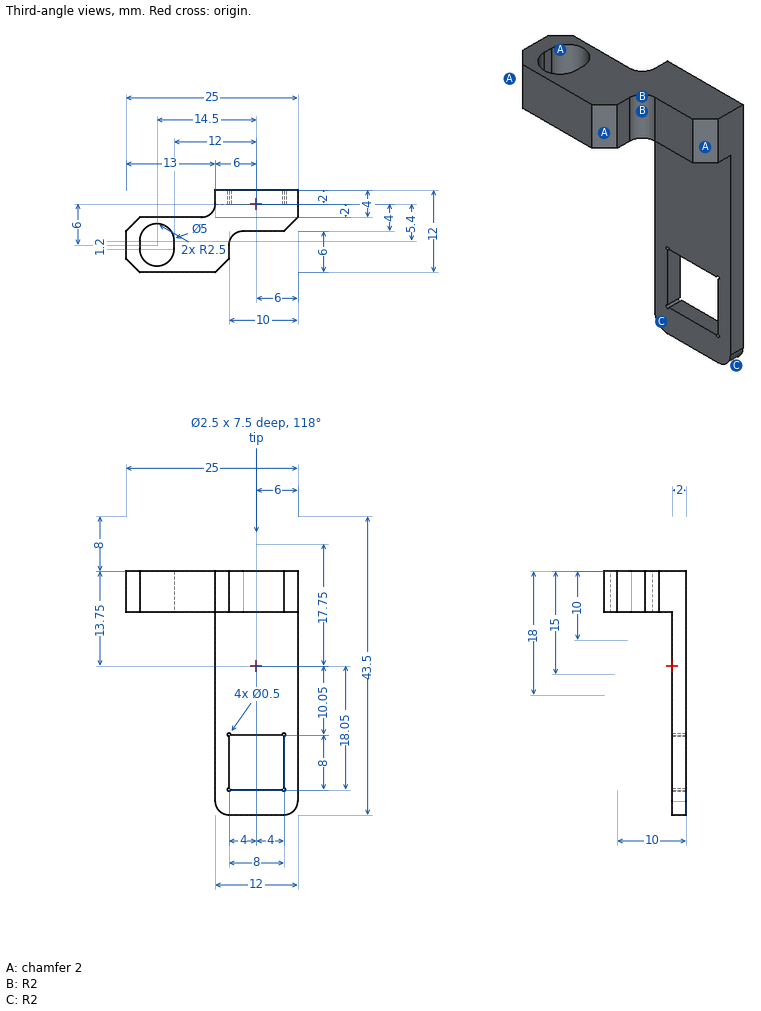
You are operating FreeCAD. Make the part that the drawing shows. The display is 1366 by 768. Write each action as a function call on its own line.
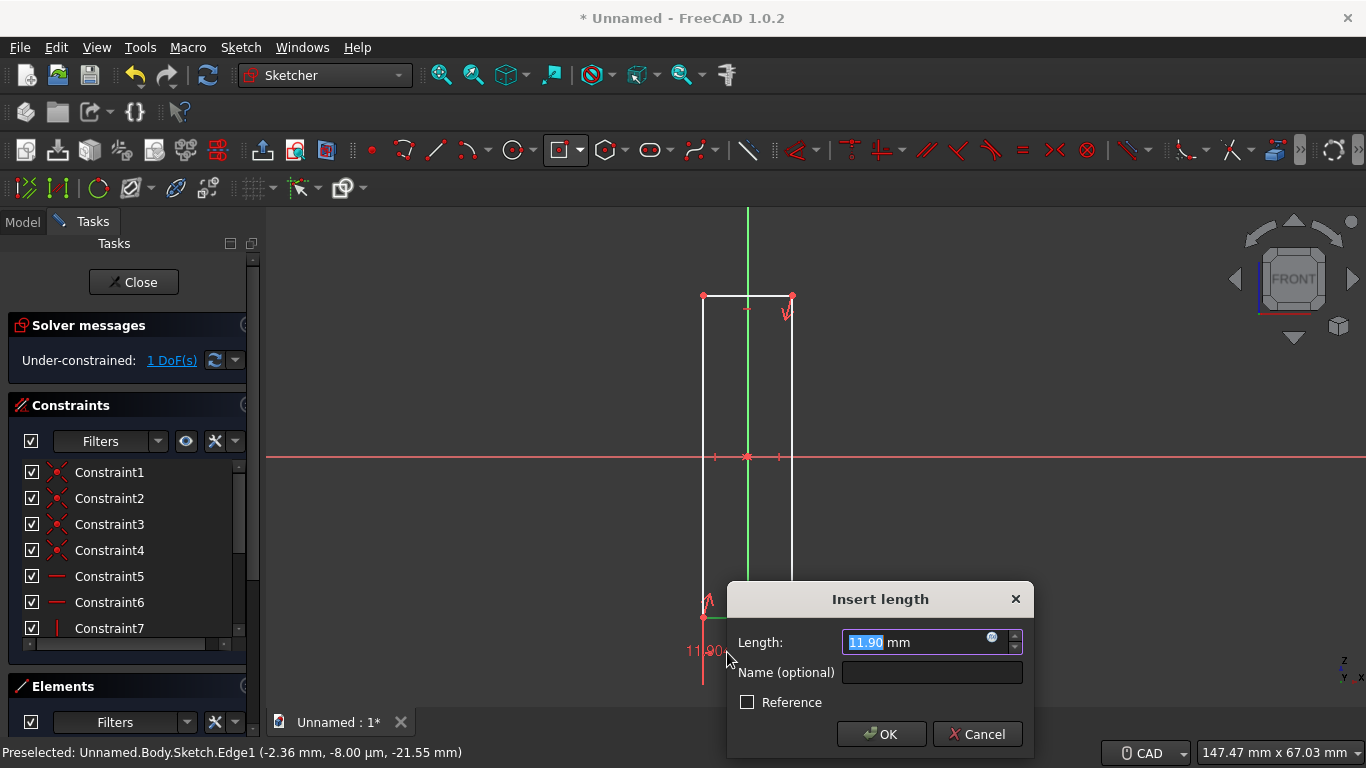
text(12)
key(Return)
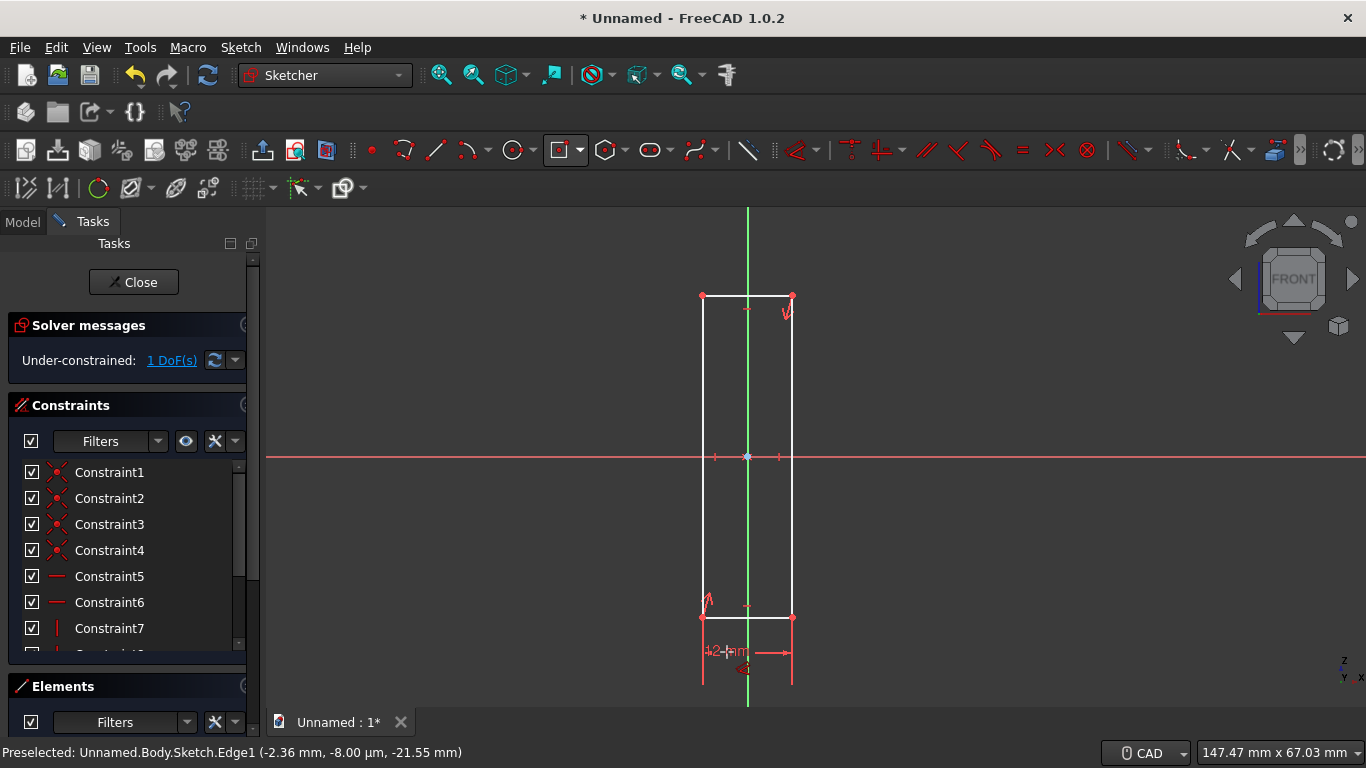
click(792, 521)
click(826, 383)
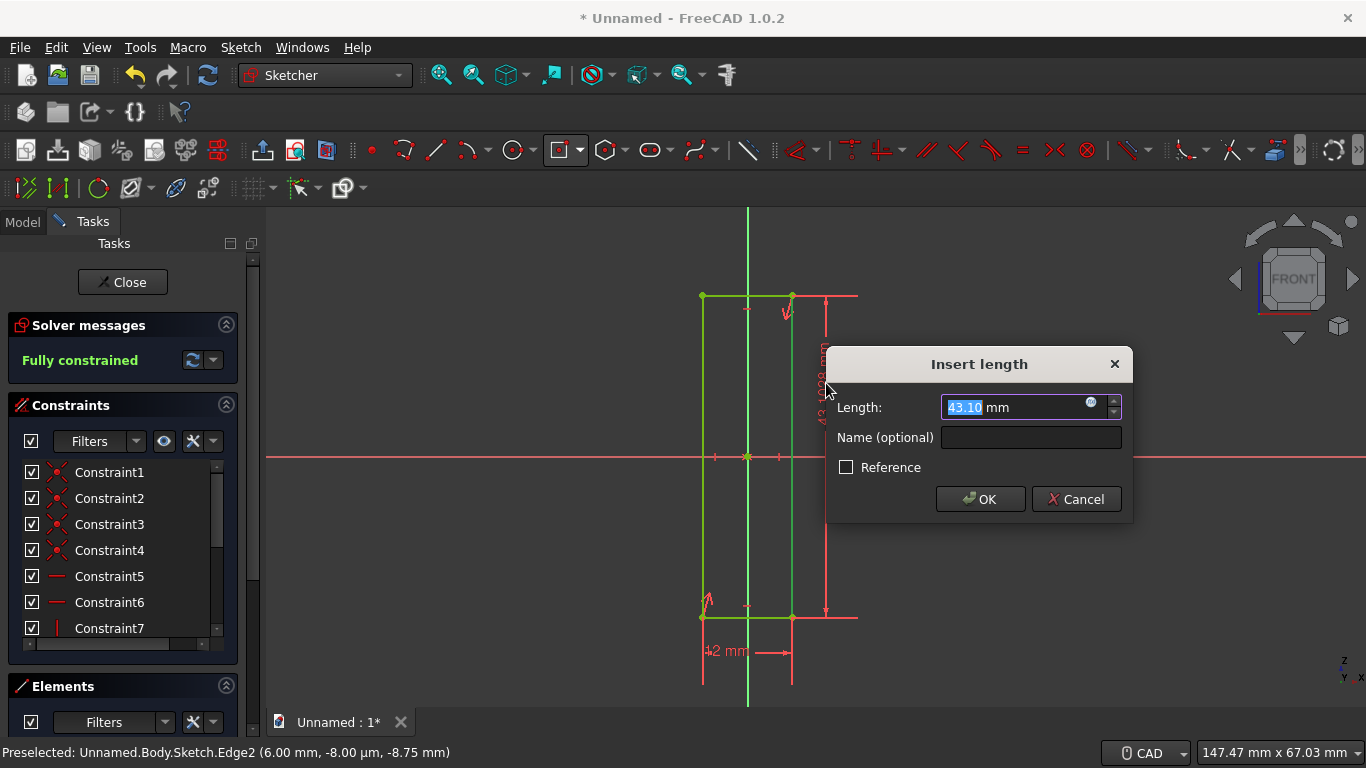
text(43.5)
key(Return)
key(Escape)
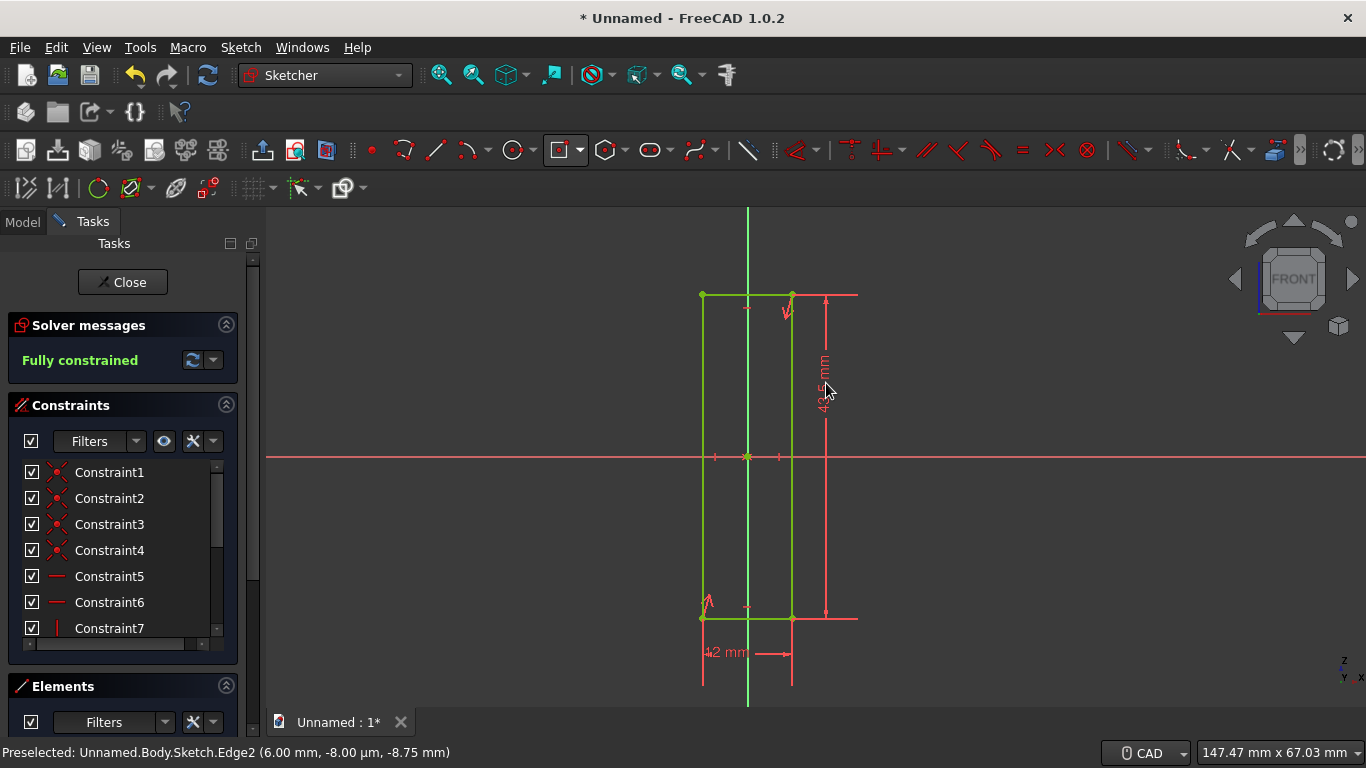
click(123, 282)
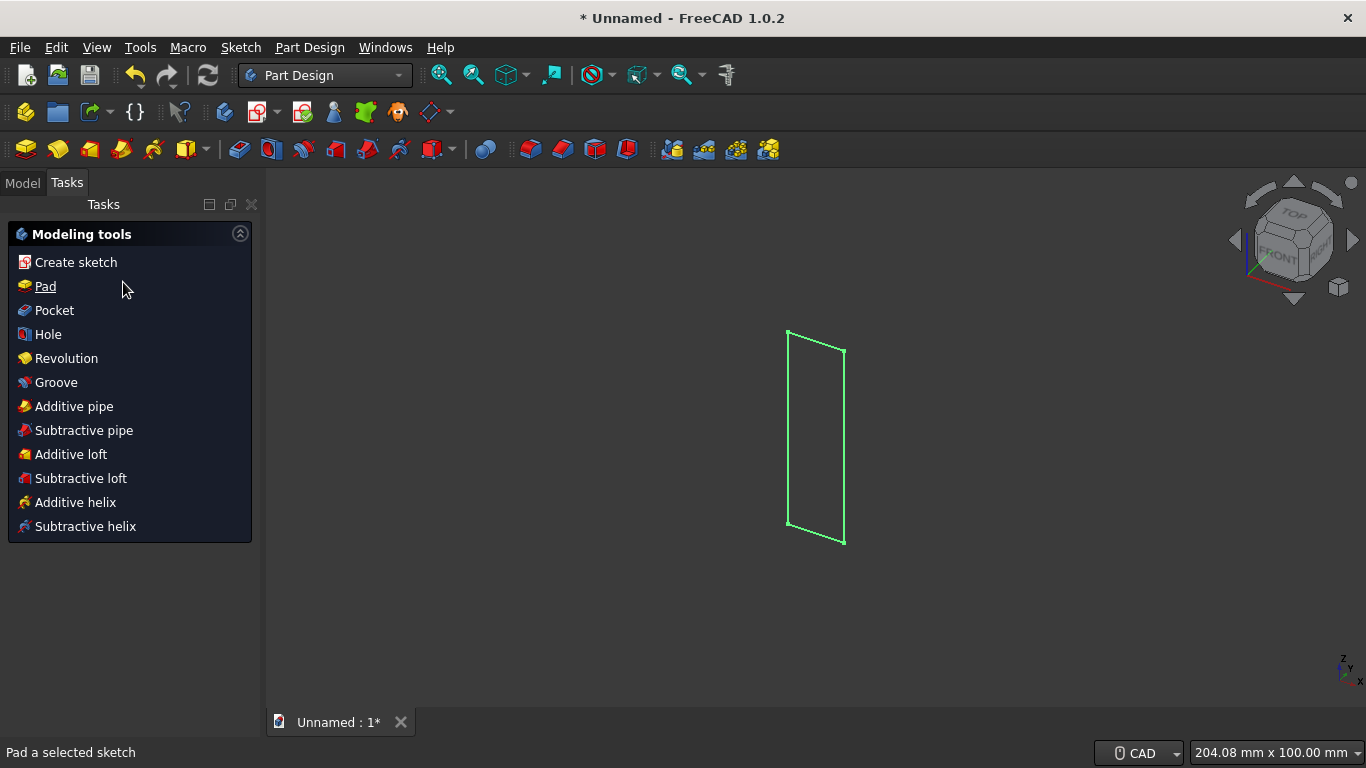
click(26, 150)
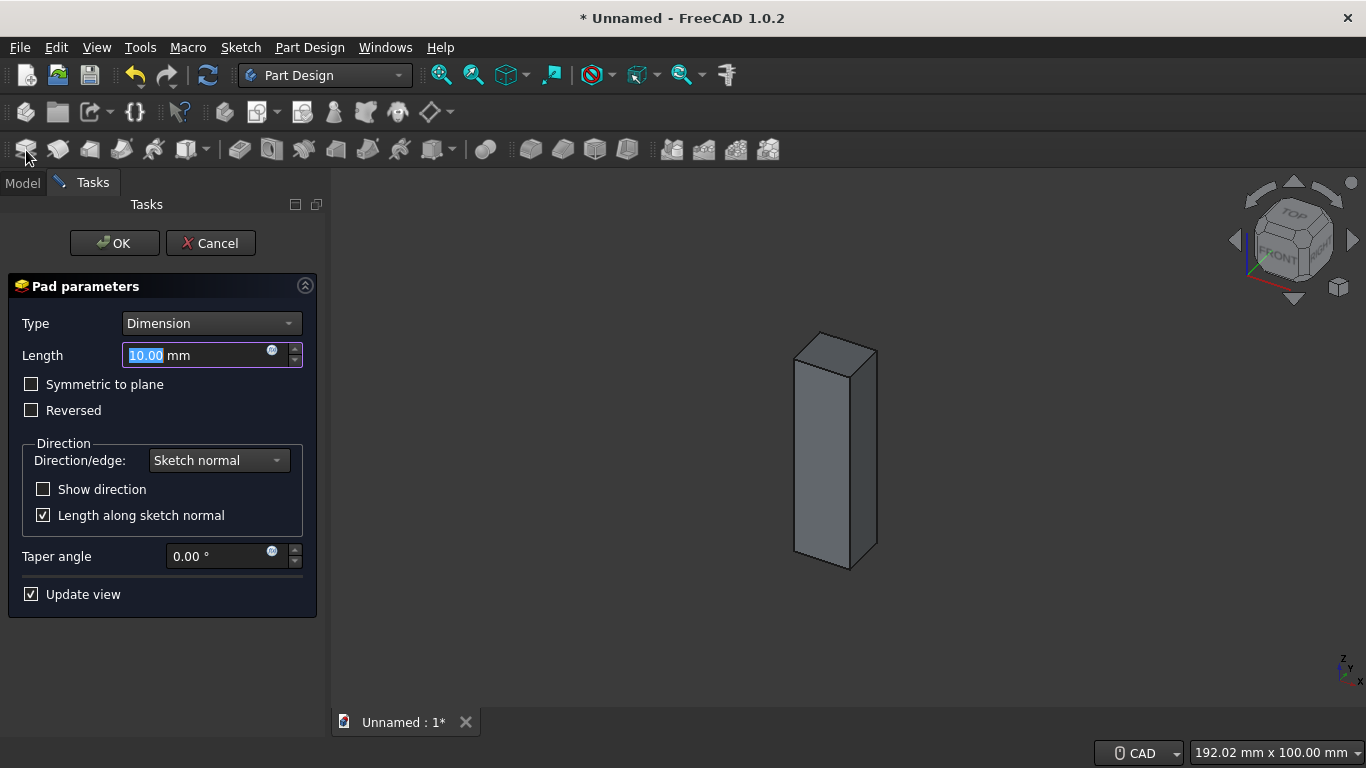
text(2)
key(Tab)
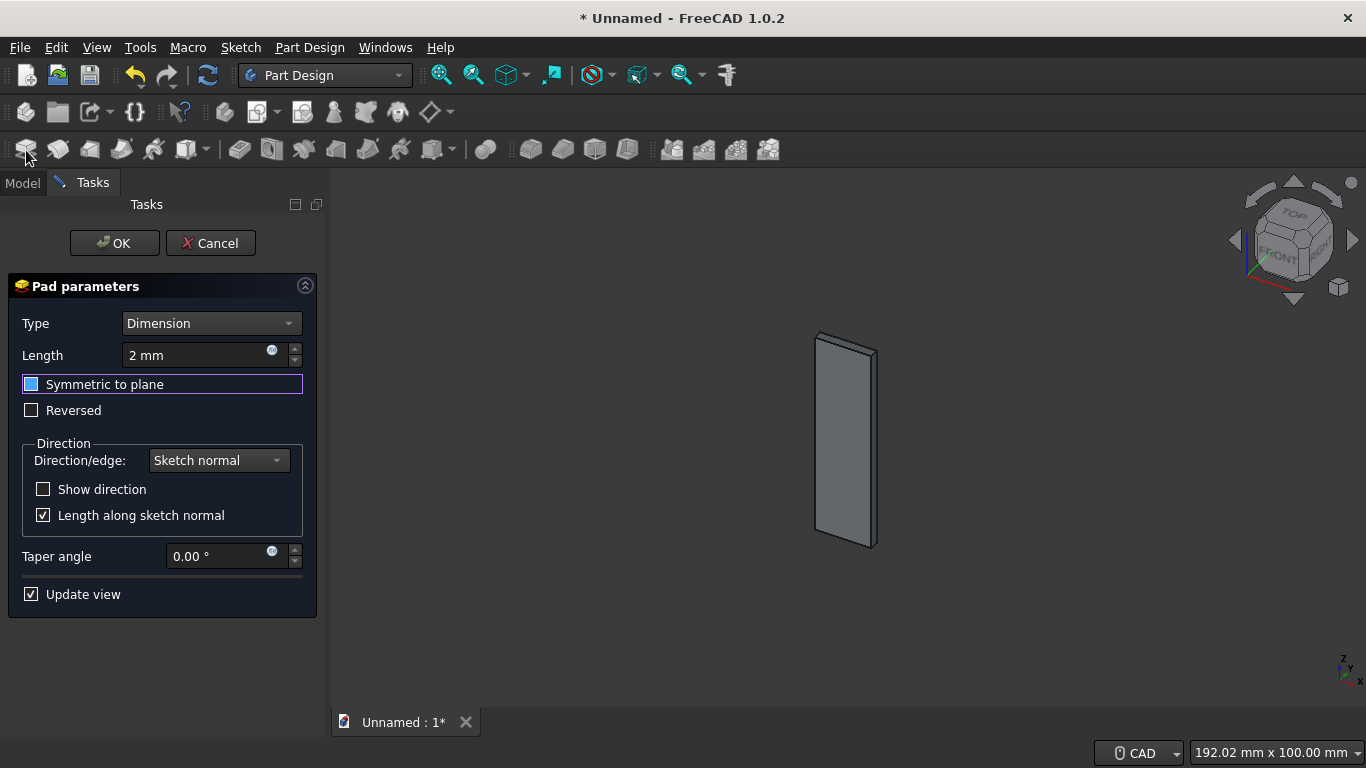
click(30, 410)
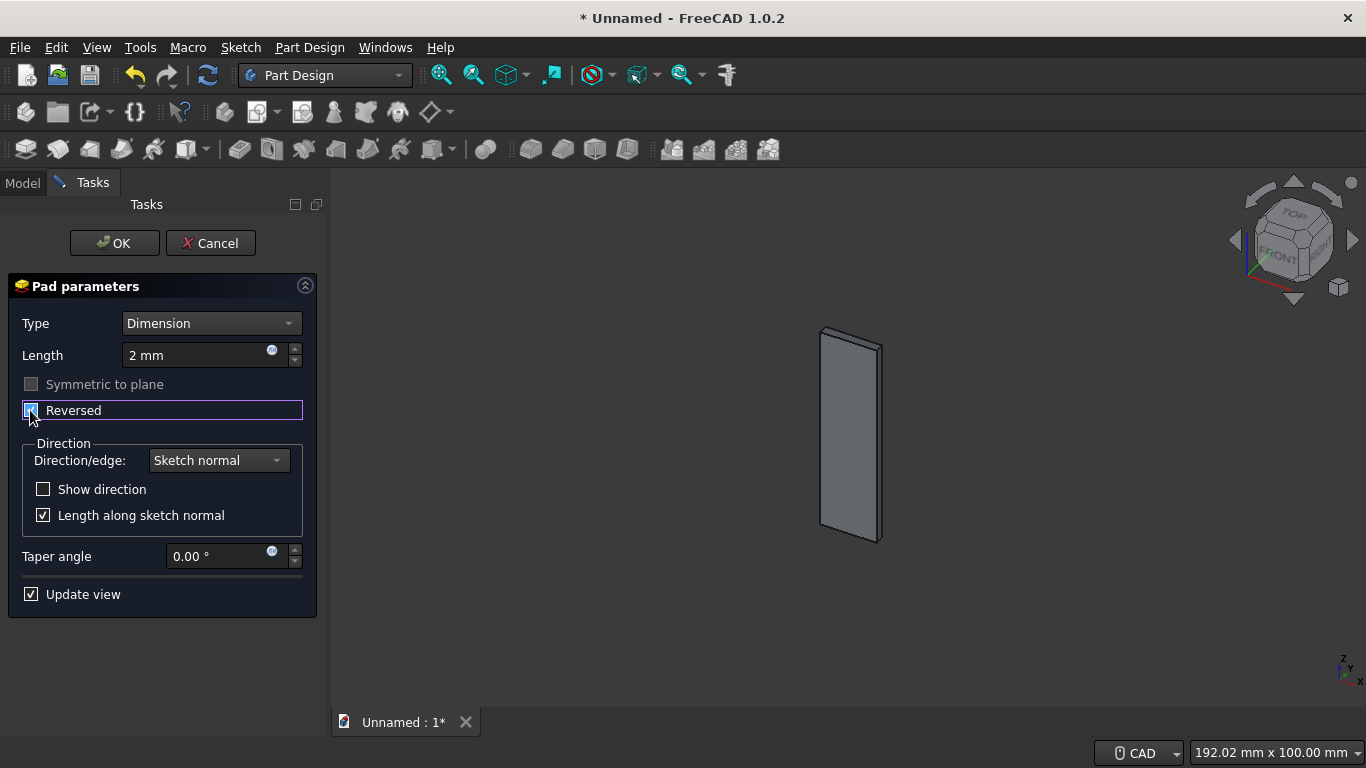
click(115, 243)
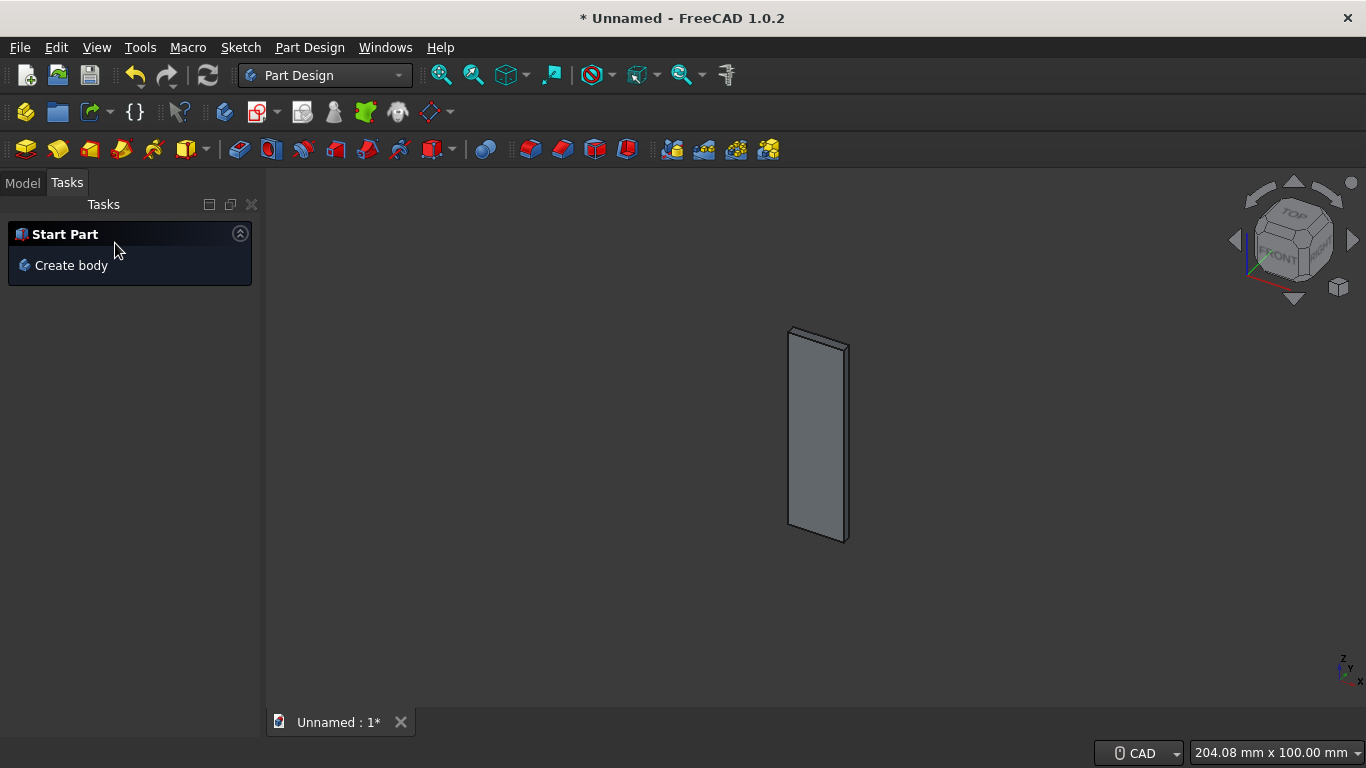
click(442, 76)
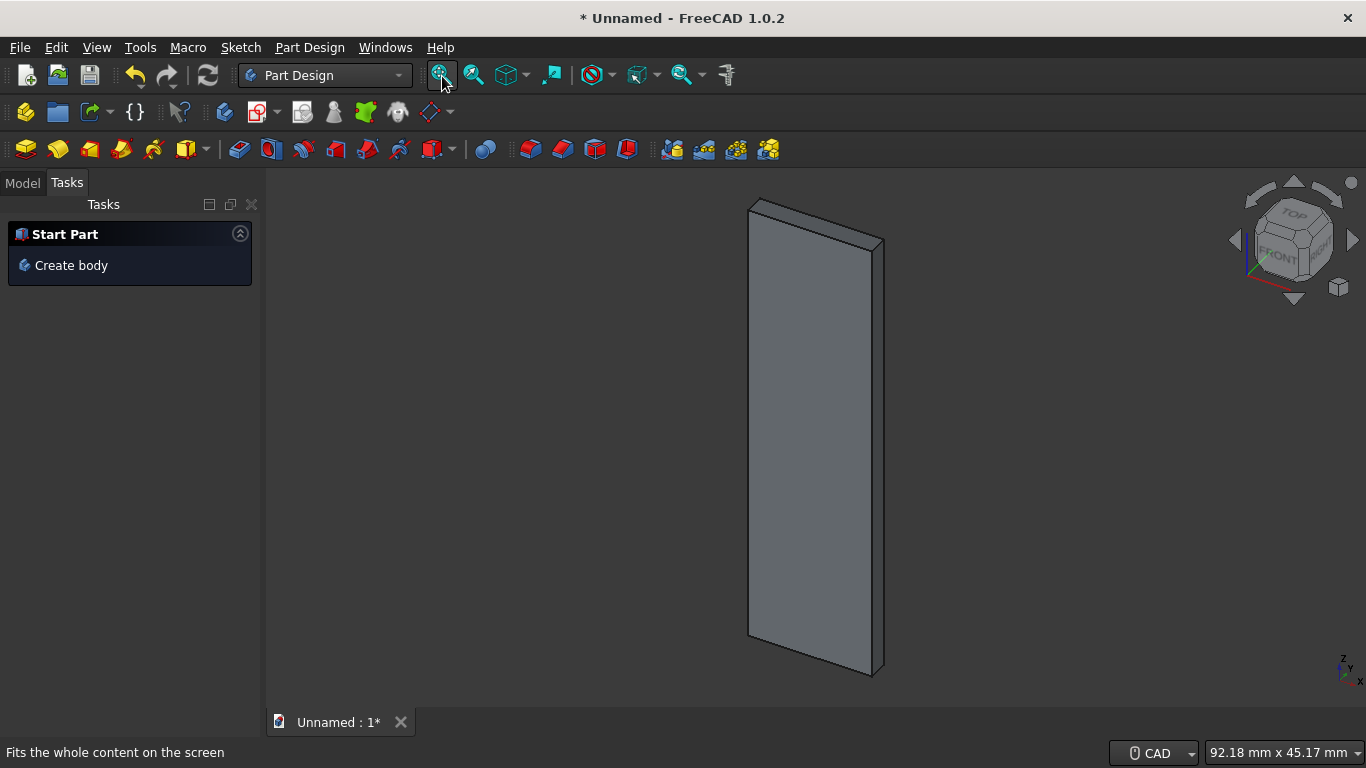
key(4)